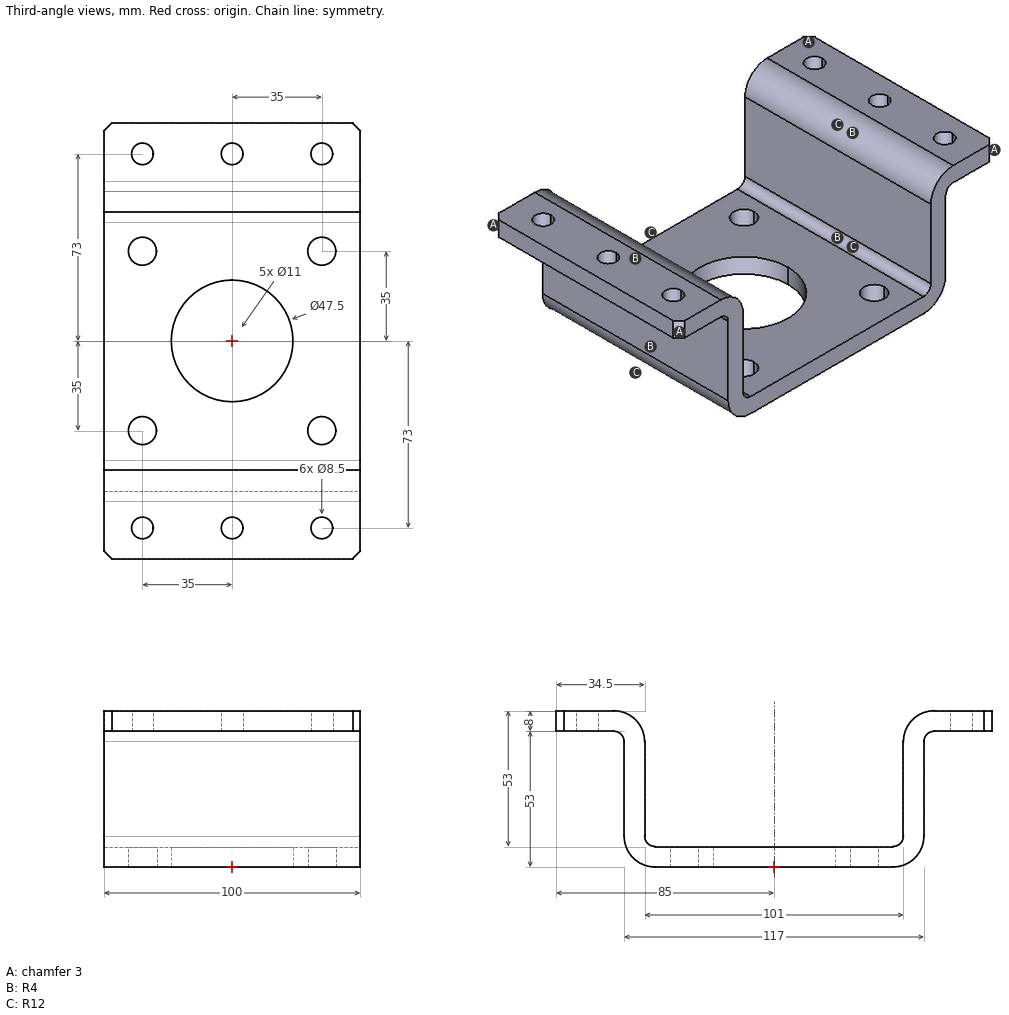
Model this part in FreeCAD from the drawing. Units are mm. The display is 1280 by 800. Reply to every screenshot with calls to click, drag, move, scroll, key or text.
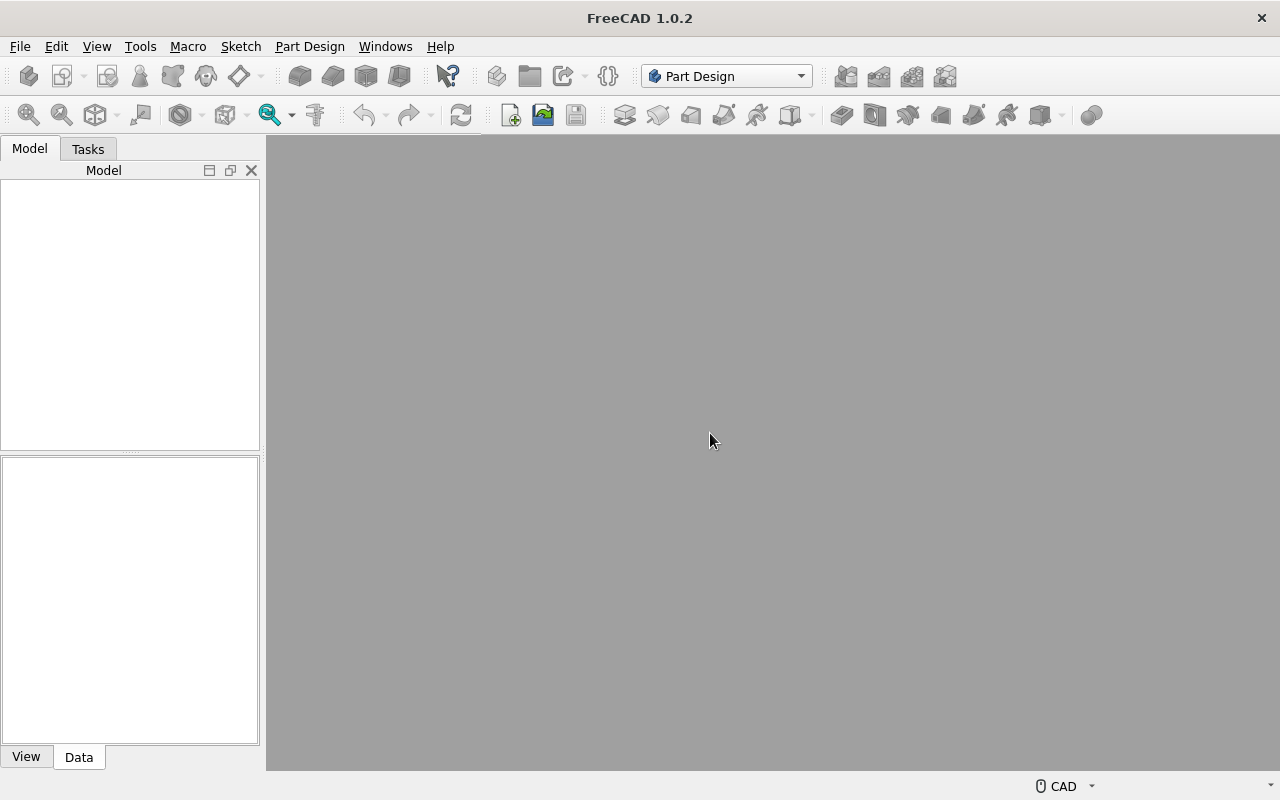
key(ctrl+n)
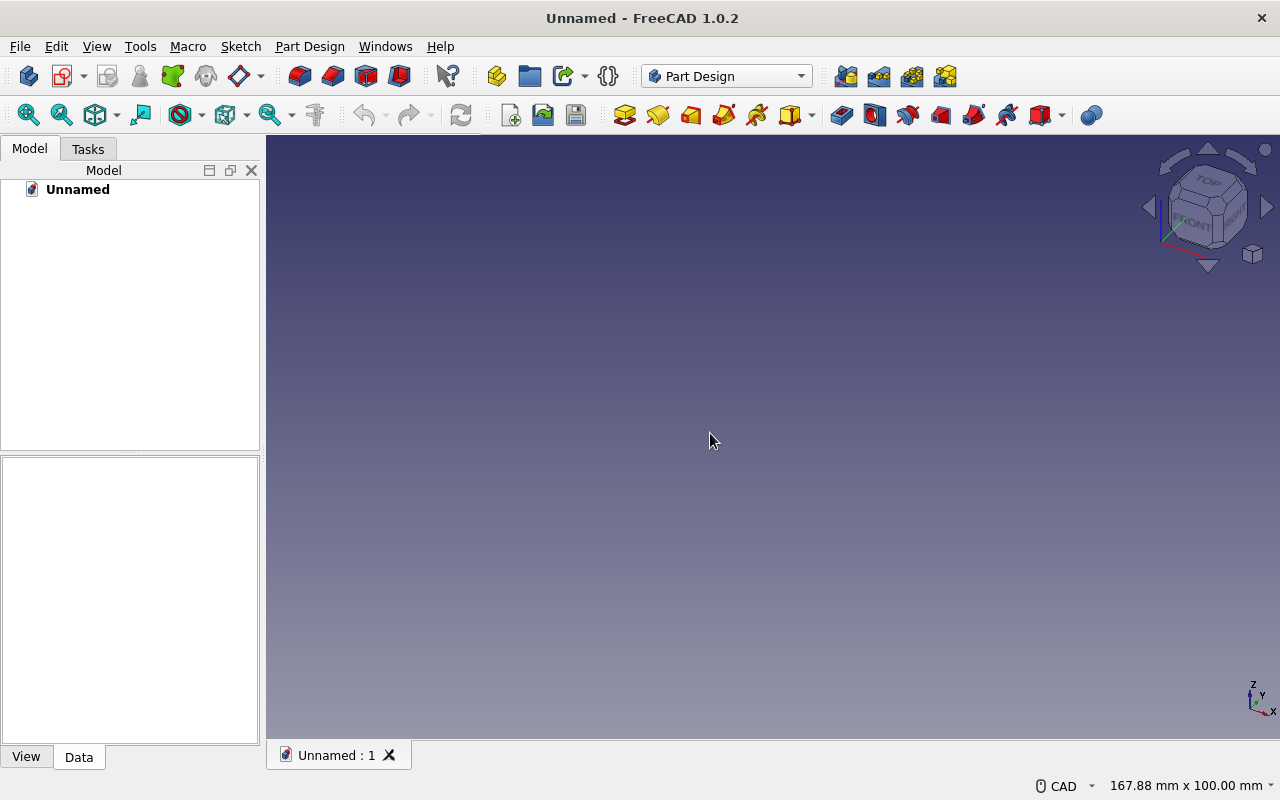
click(62, 76)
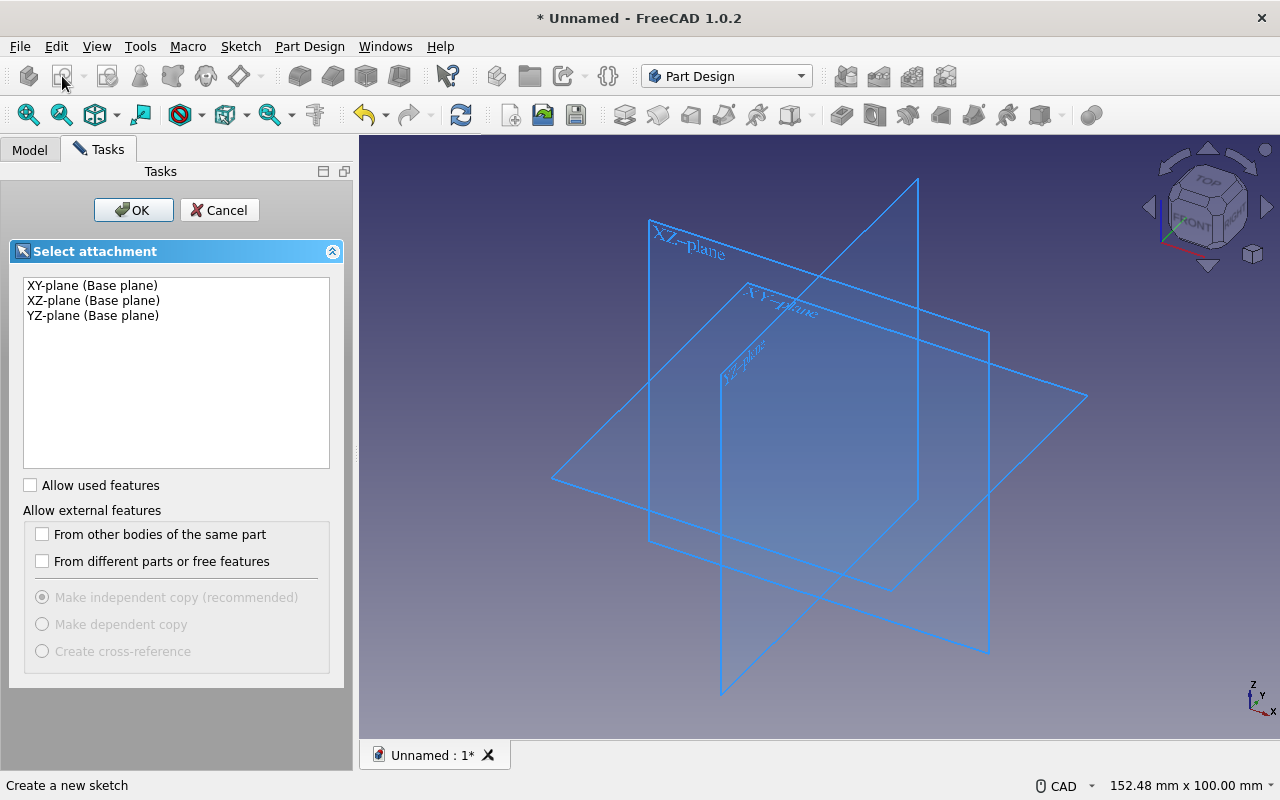
click(84, 316)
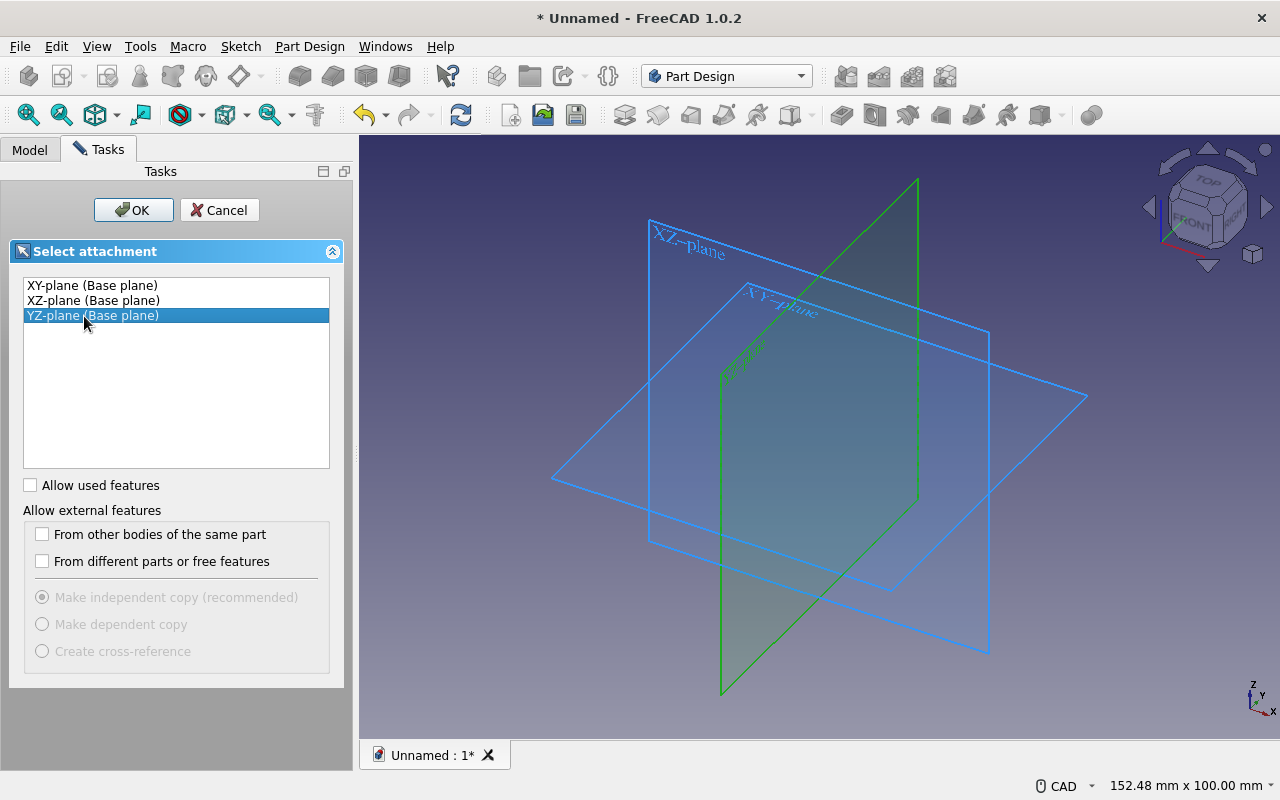
click(134, 210)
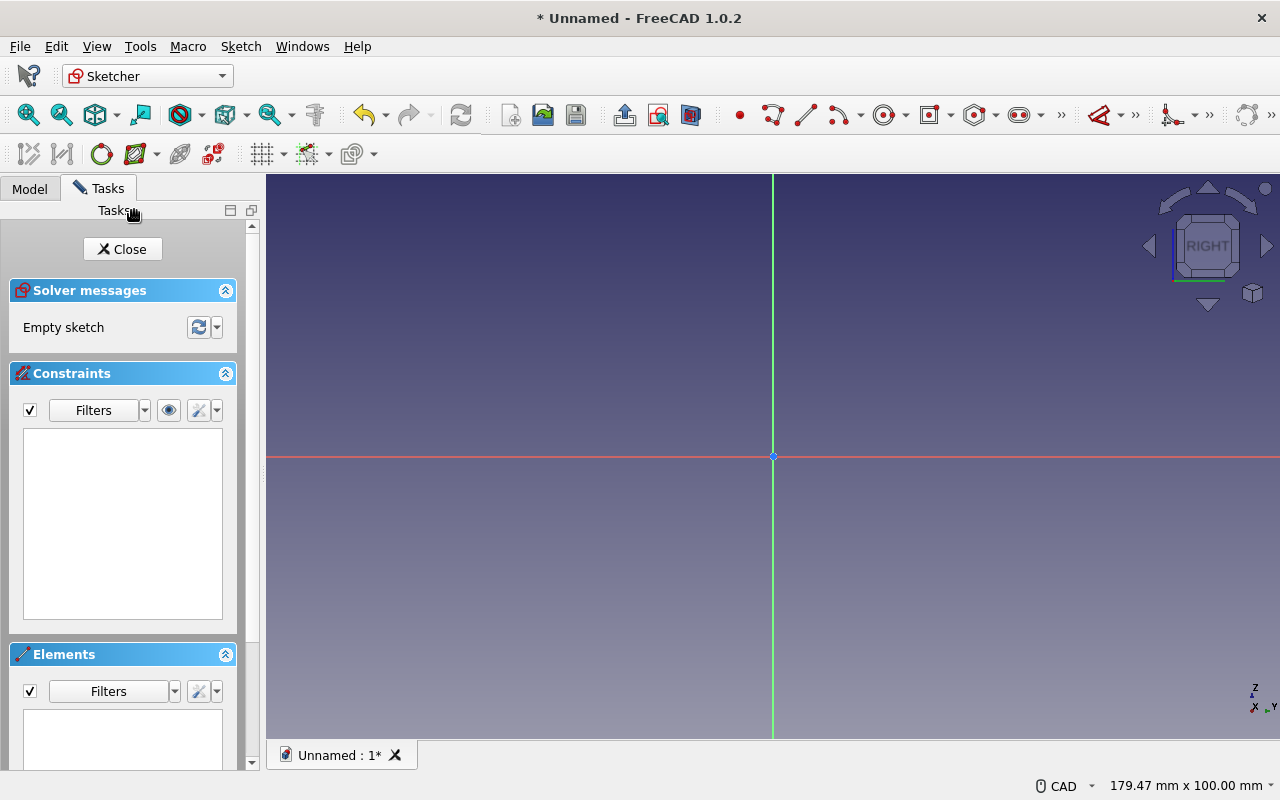
scroll(621, 666, down, 3)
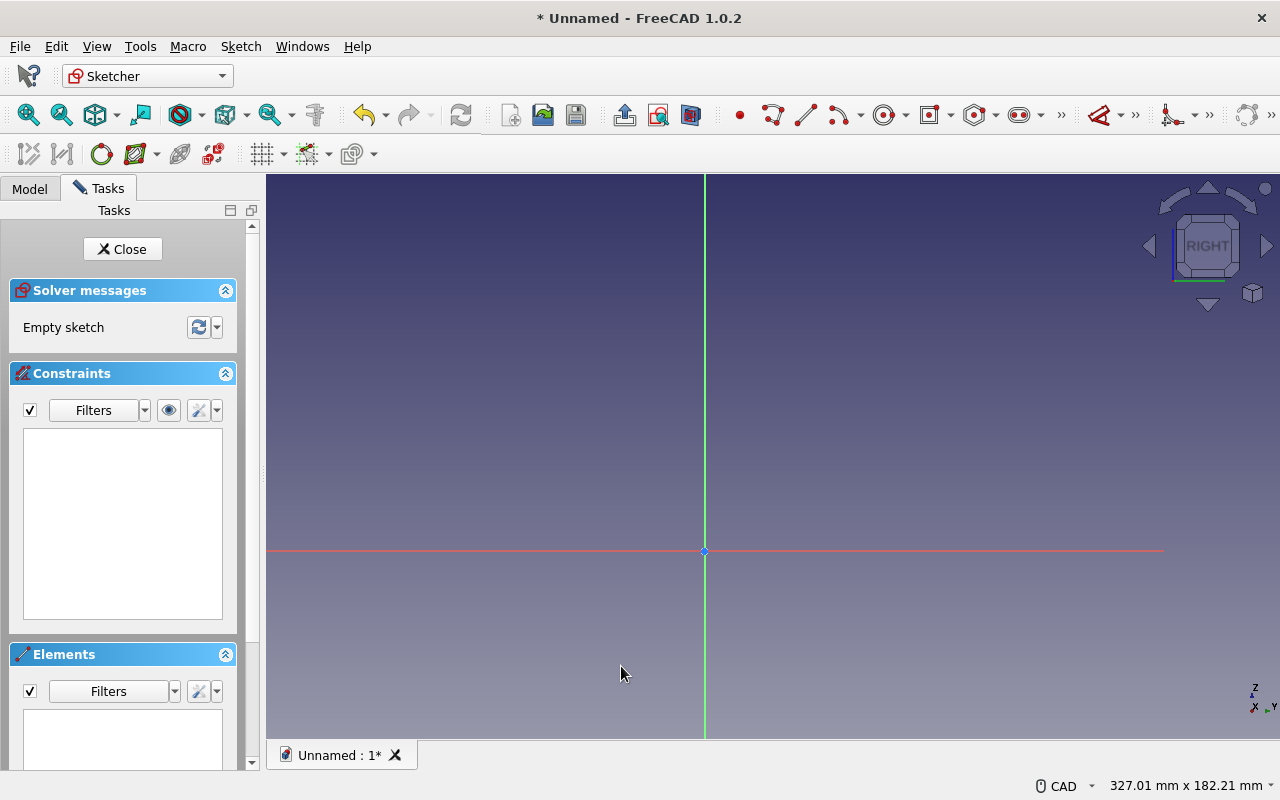
key(g)
key(m)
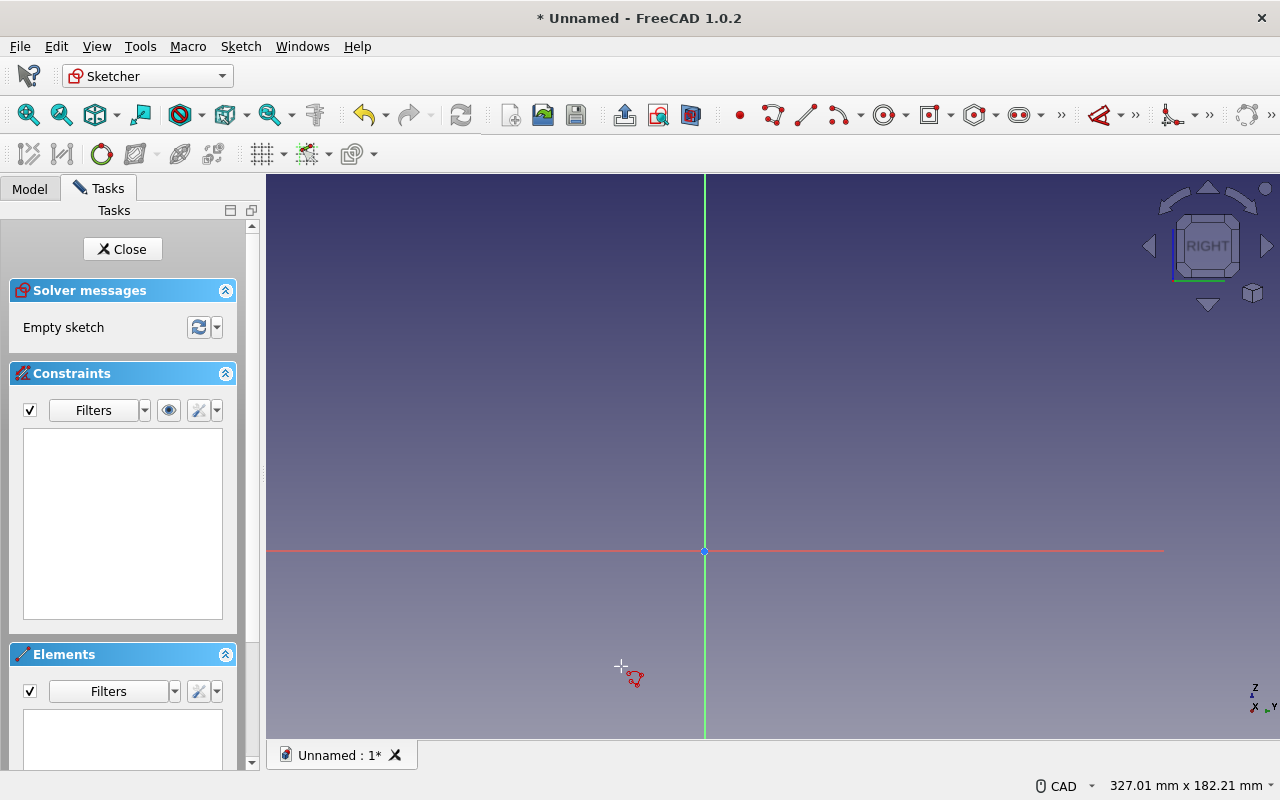
click(861, 527)
click(548, 527)
click(548, 362)
click(441, 362)
click(441, 387)
click(523, 387)
click(523, 551)
click(886, 542)
click(886, 387)
click(968, 387)
click(968, 362)
click(861, 362)
click(861, 528)
key(Escape)
key(Escape)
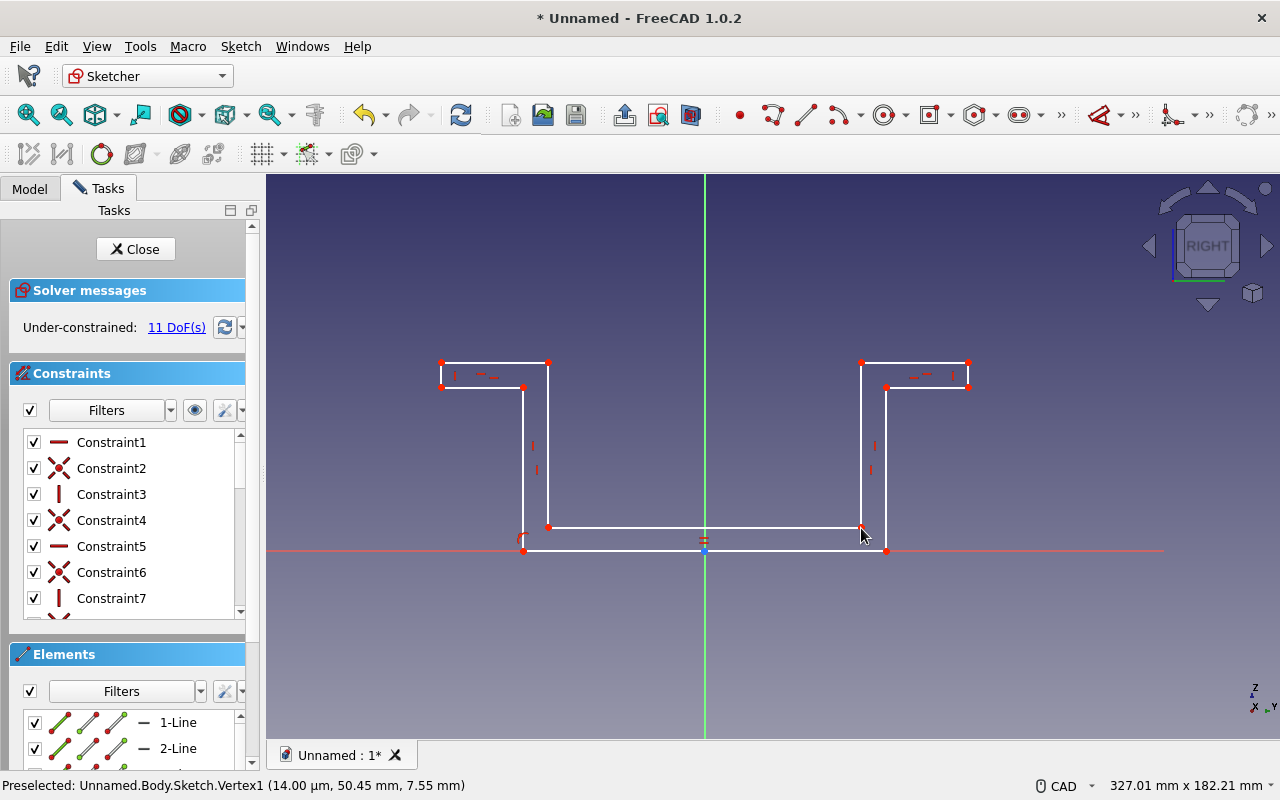
click(523, 388)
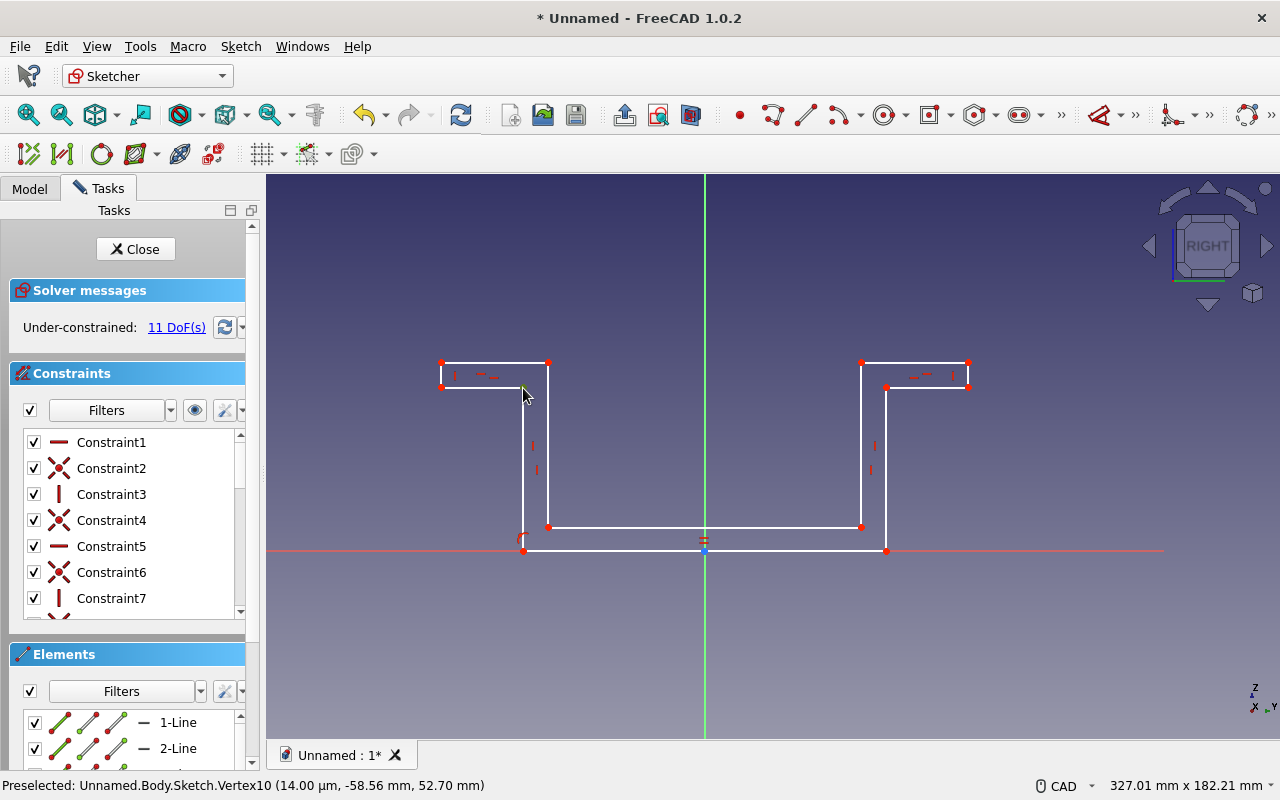
click(886, 388)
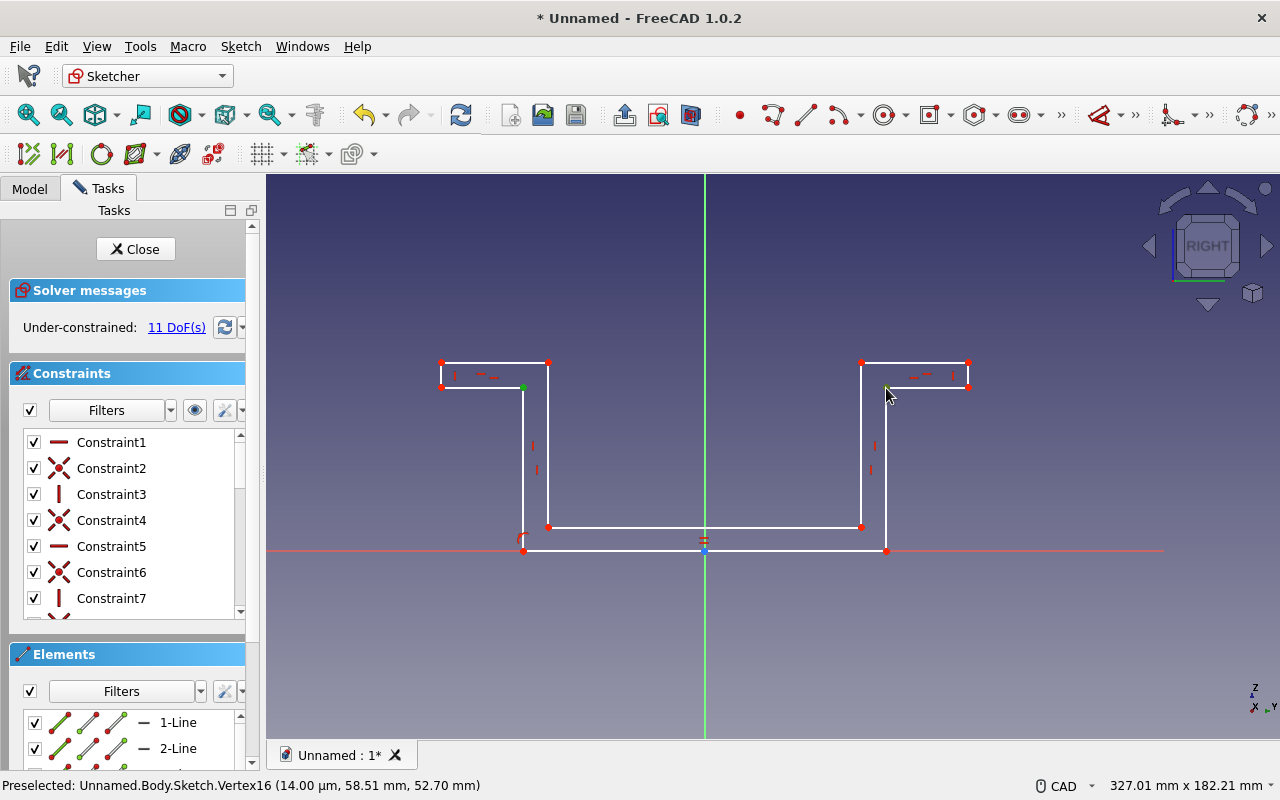
click(705, 675)